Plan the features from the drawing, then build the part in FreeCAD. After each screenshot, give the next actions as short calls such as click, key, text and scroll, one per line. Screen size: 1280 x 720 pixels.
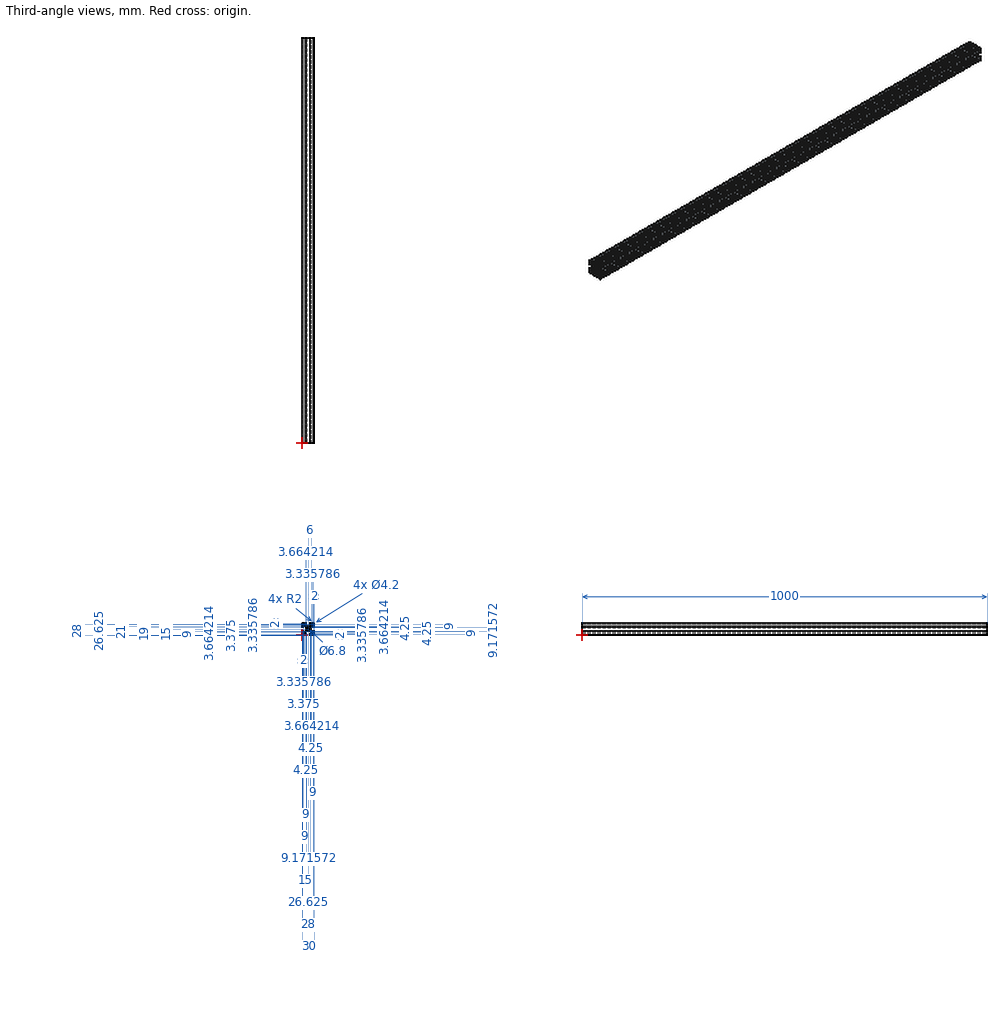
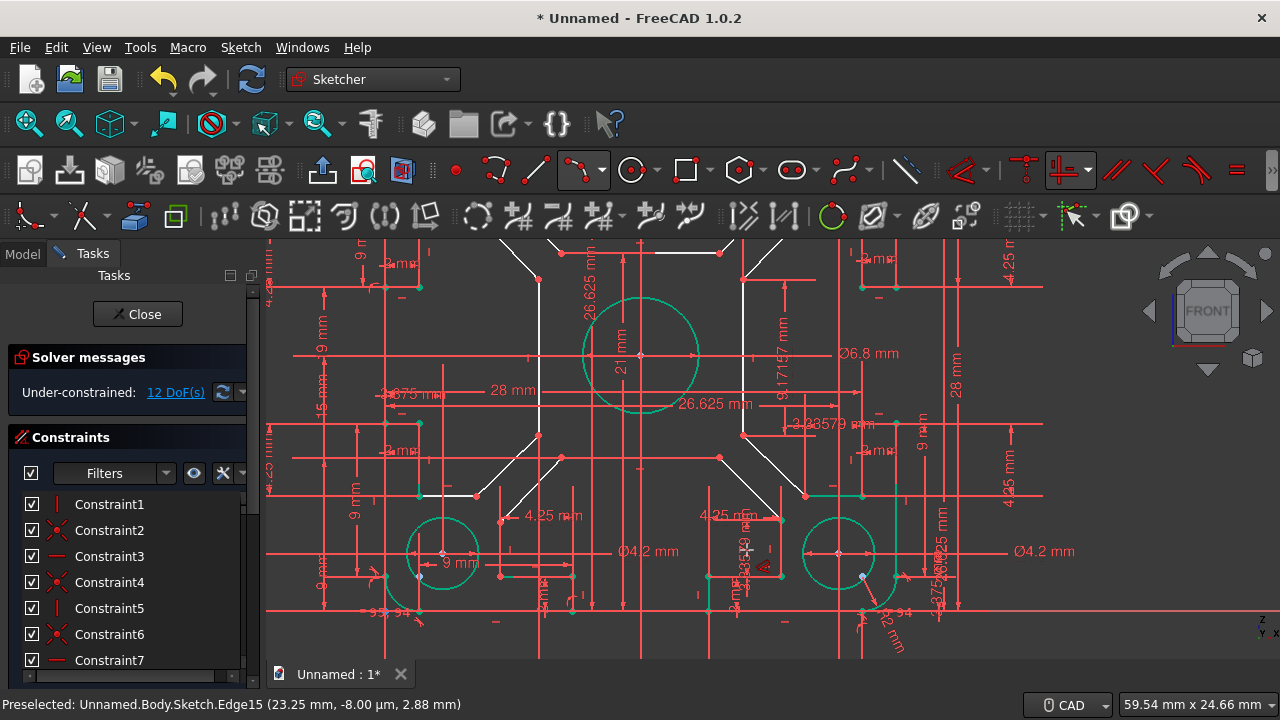
click(672, 458)
click(641, 492)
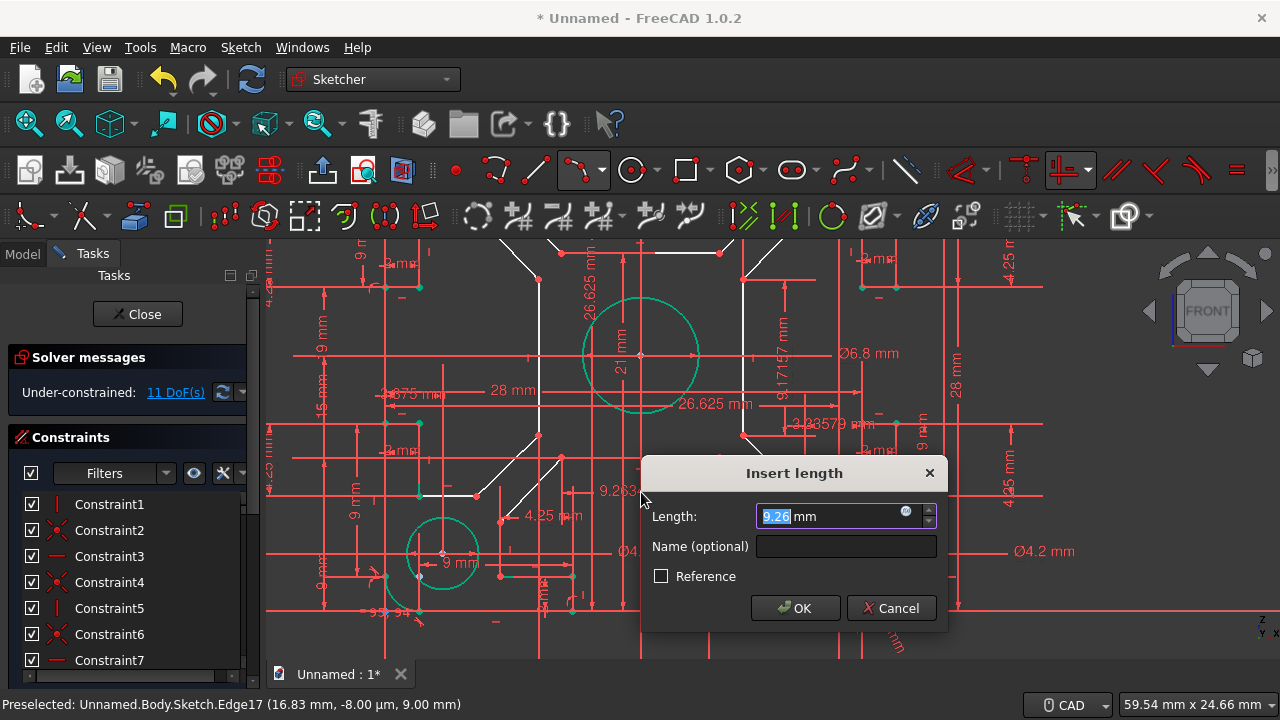
text(9.171572)
key(Return)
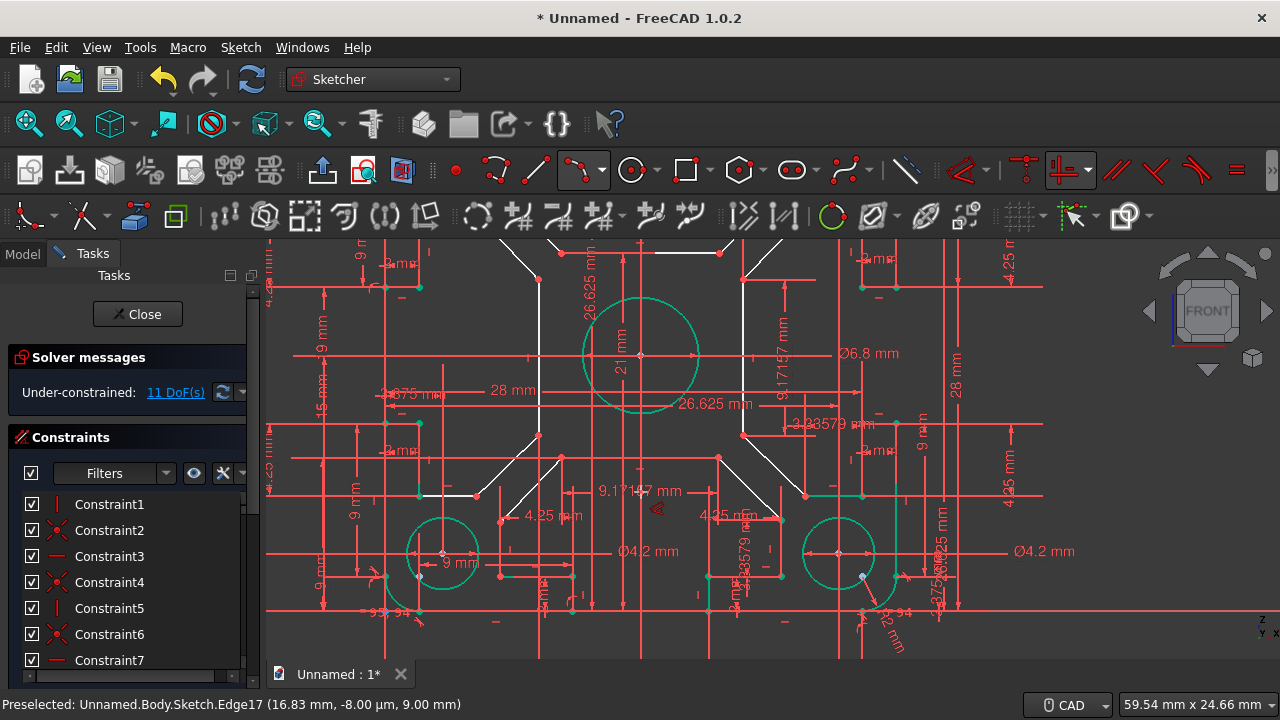
click(500, 539)
click(534, 550)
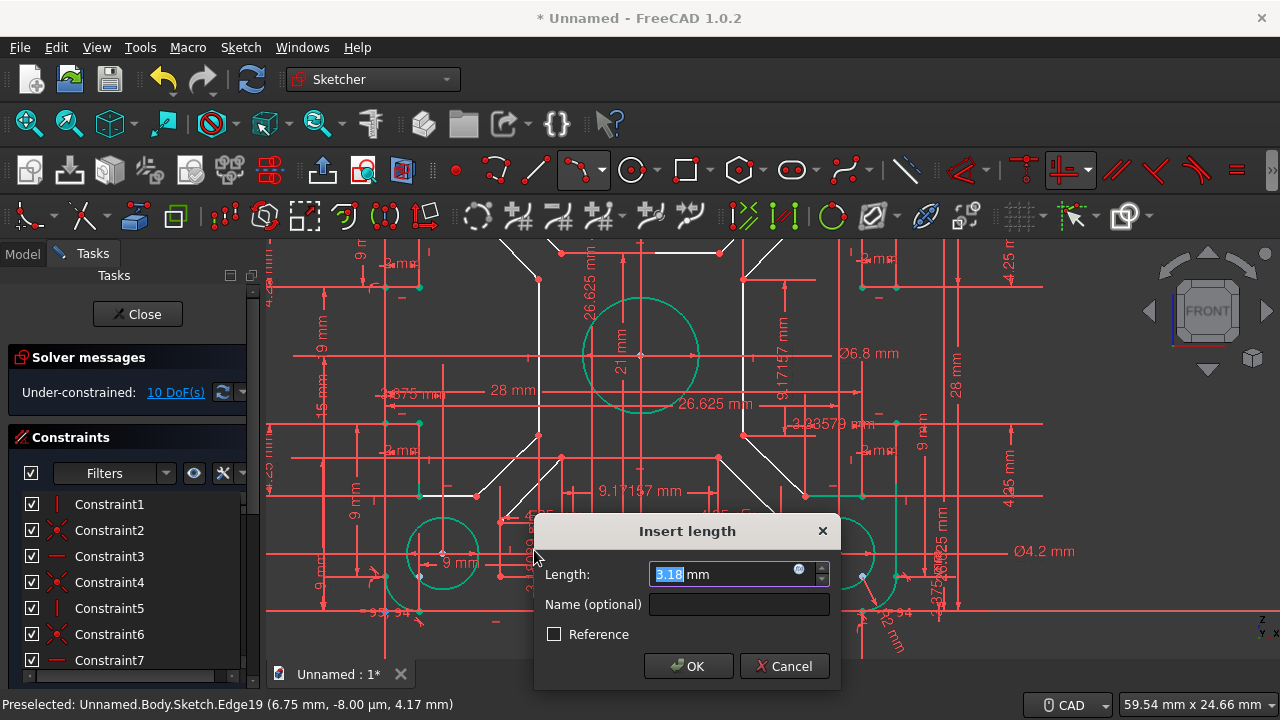
text(3.335786)
key(Return)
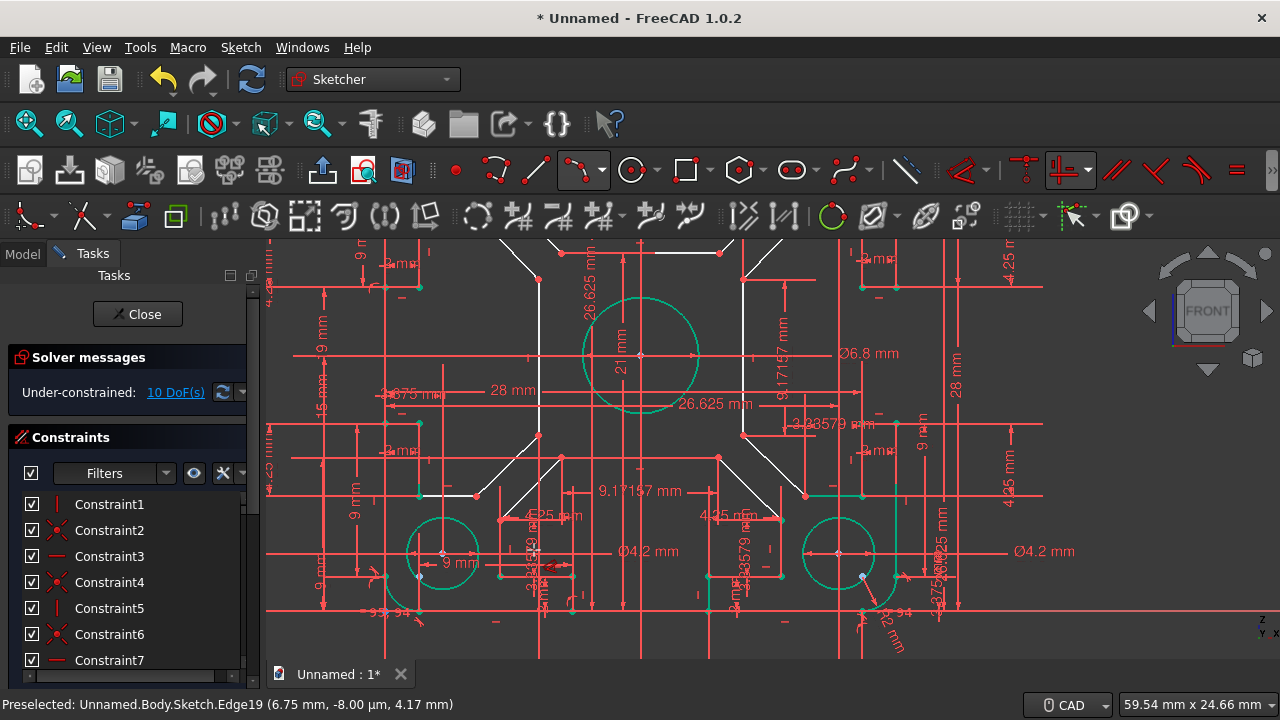
click(437, 496)
click(448, 626)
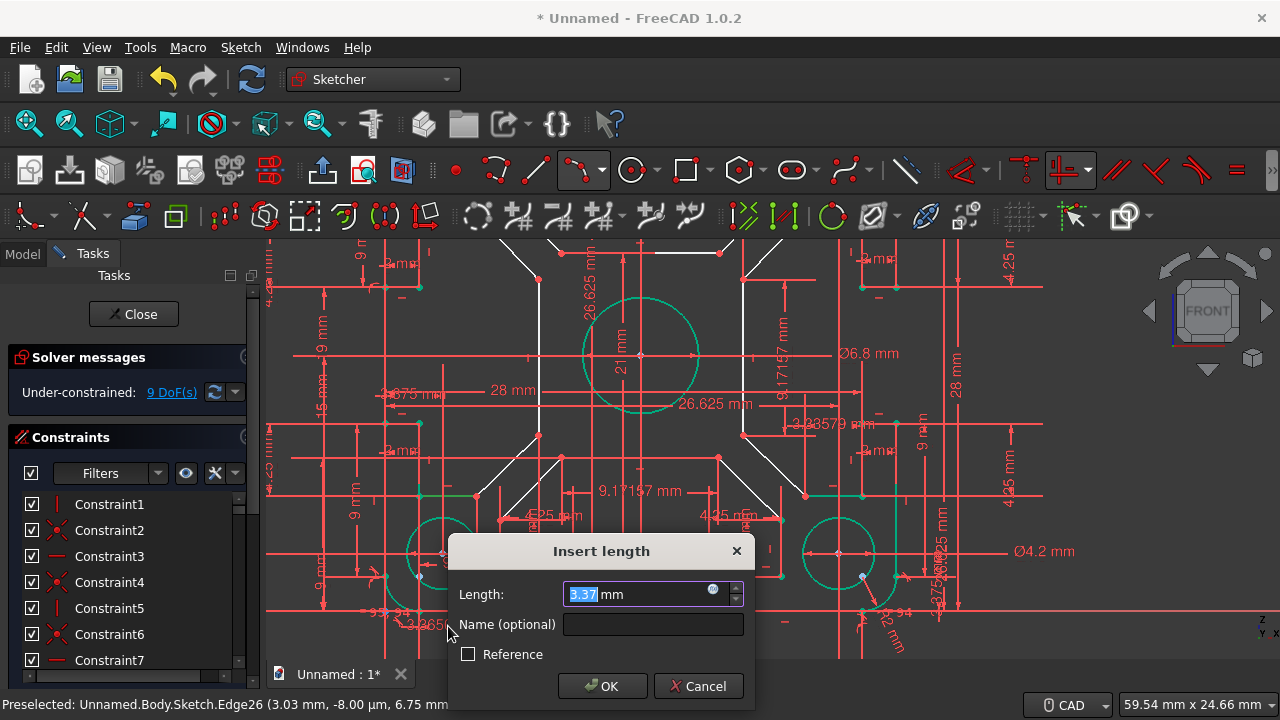
text(3.335786)
key(Return)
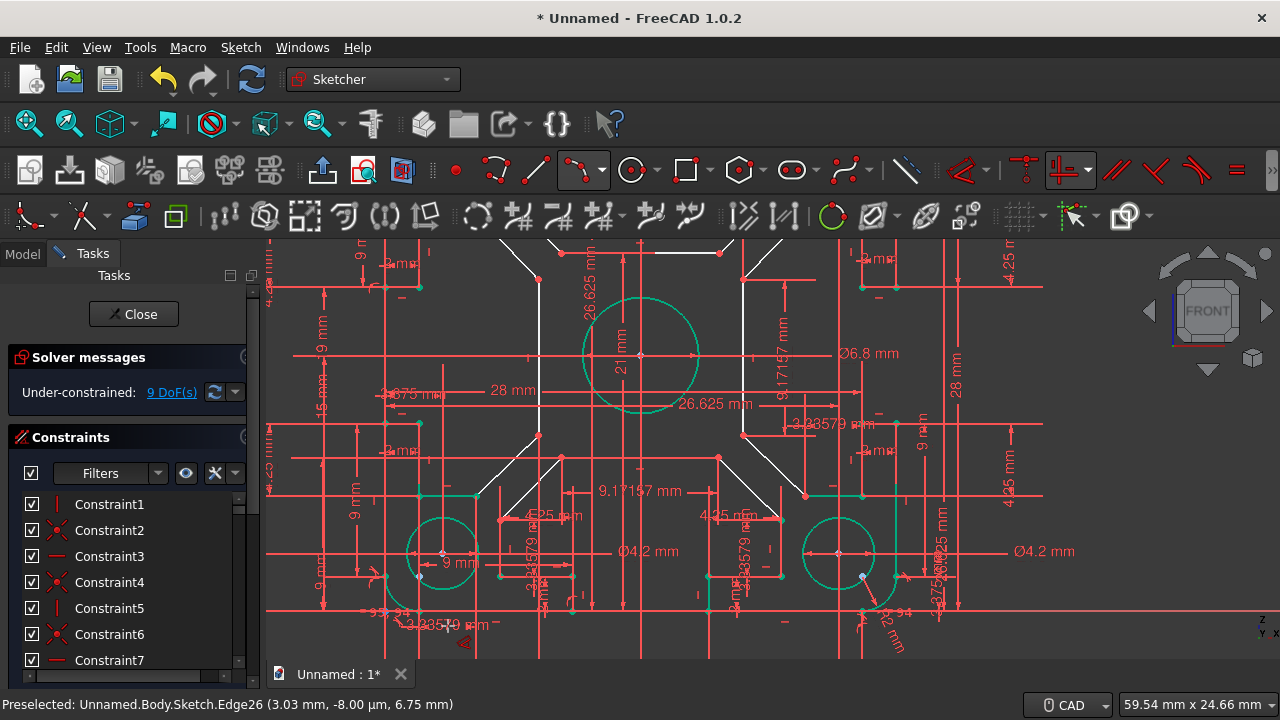
click(539, 389)
click(505, 358)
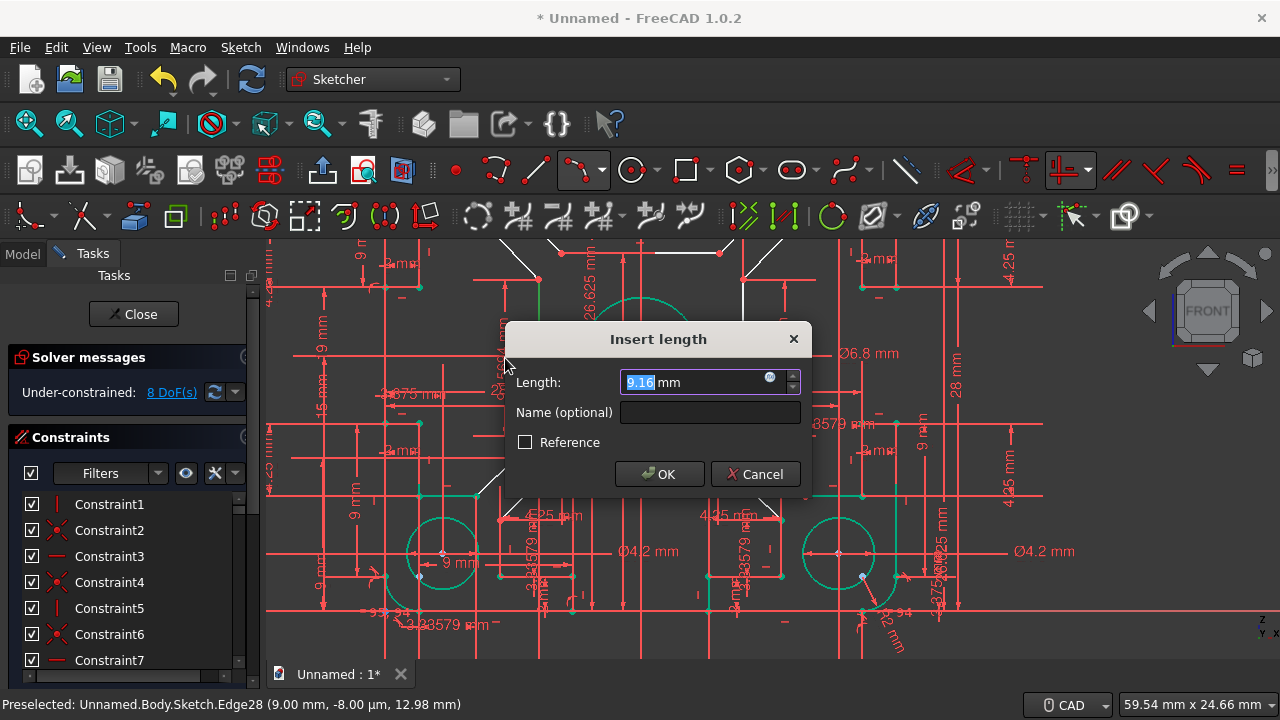
text(9.171572)
key(Return)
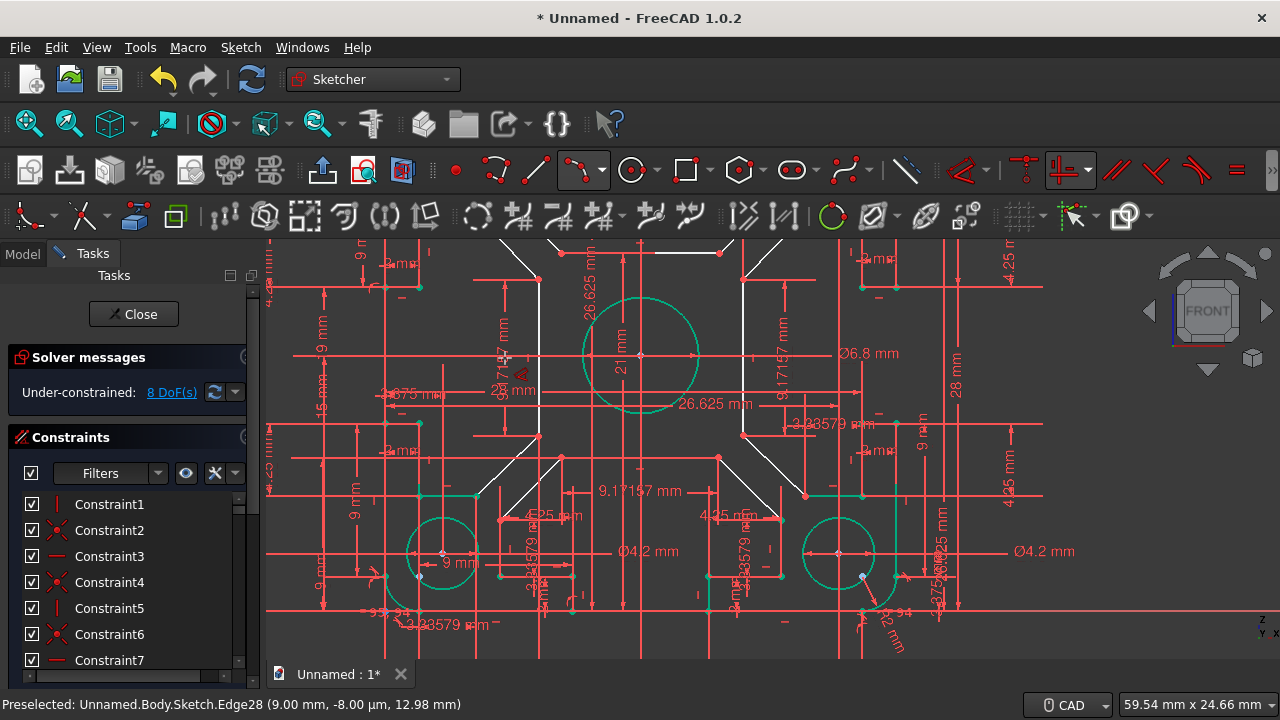
scroll(782, 563, down, 3)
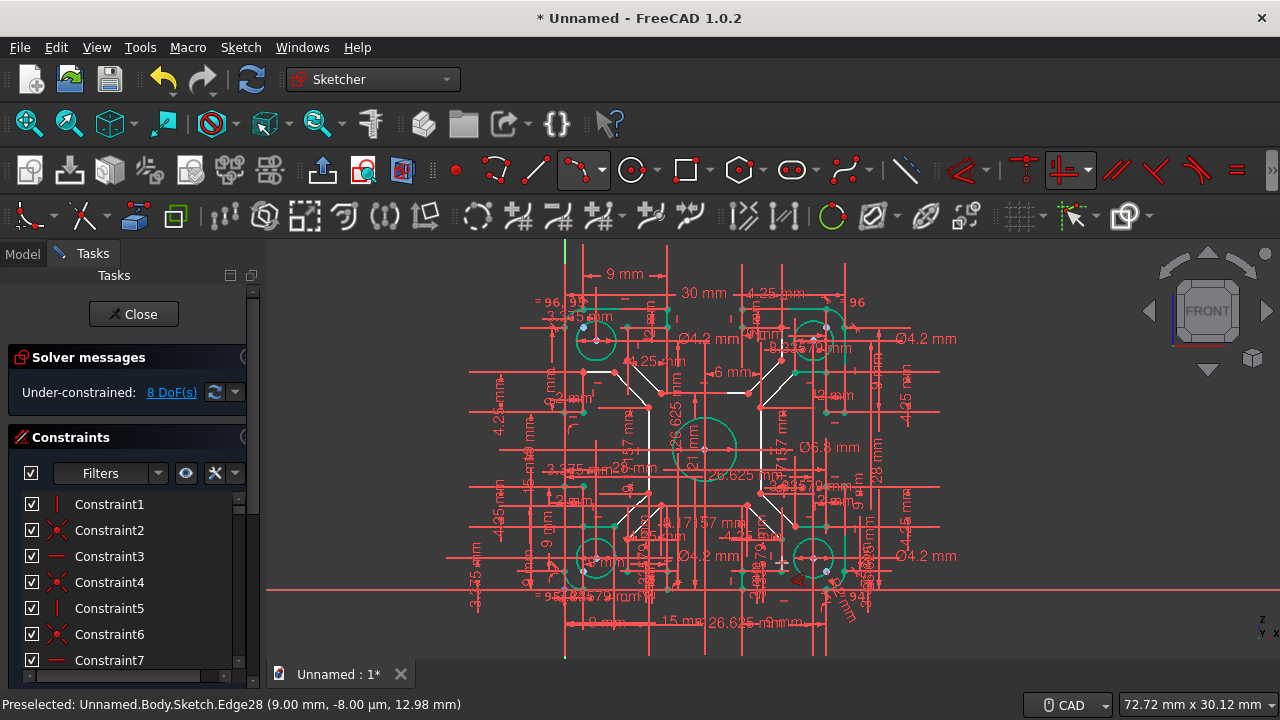
scroll(605, 372, up, 2)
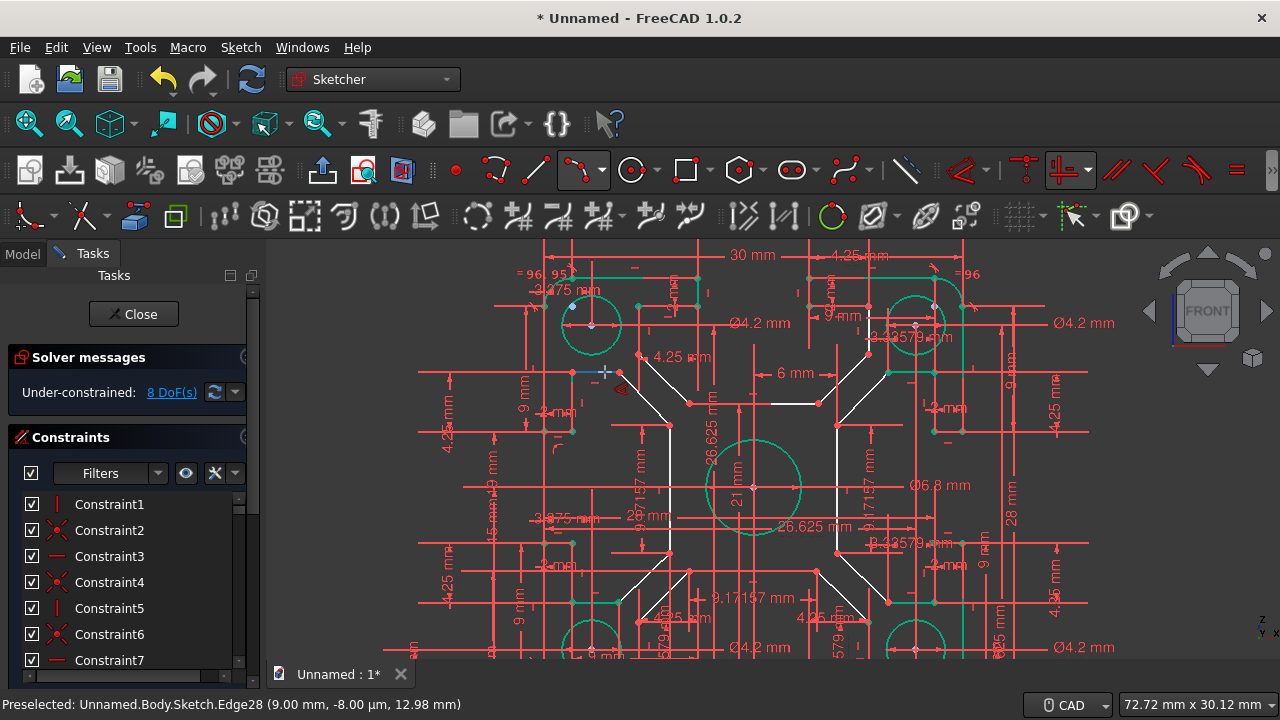
click(605, 372)
click(596, 338)